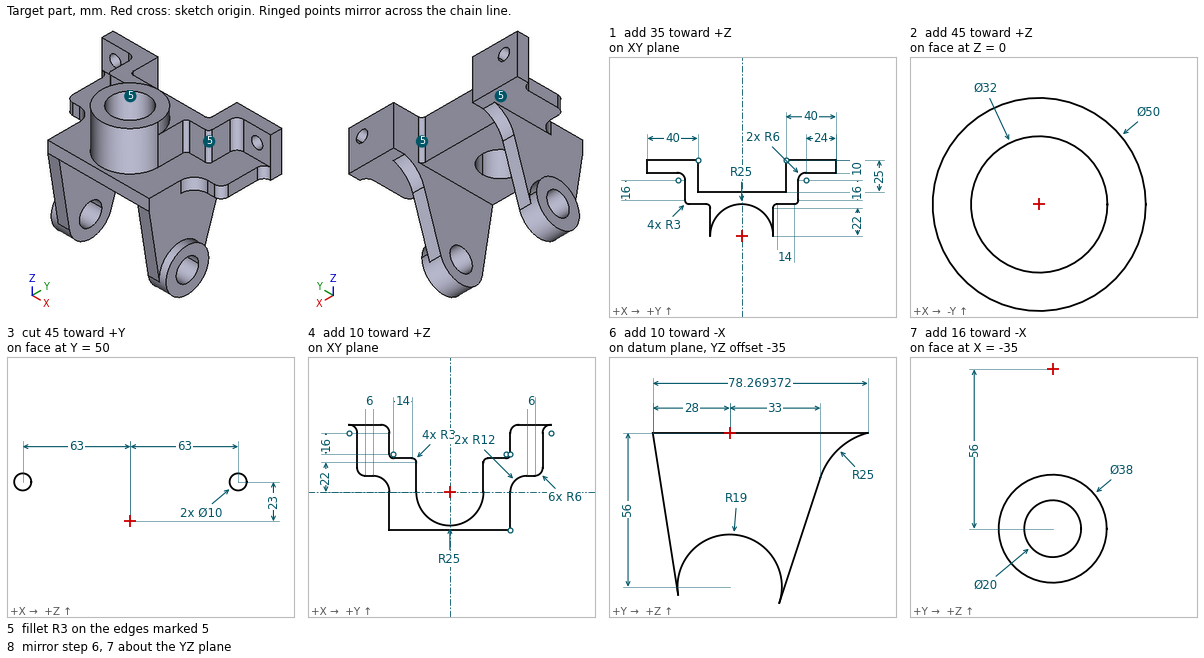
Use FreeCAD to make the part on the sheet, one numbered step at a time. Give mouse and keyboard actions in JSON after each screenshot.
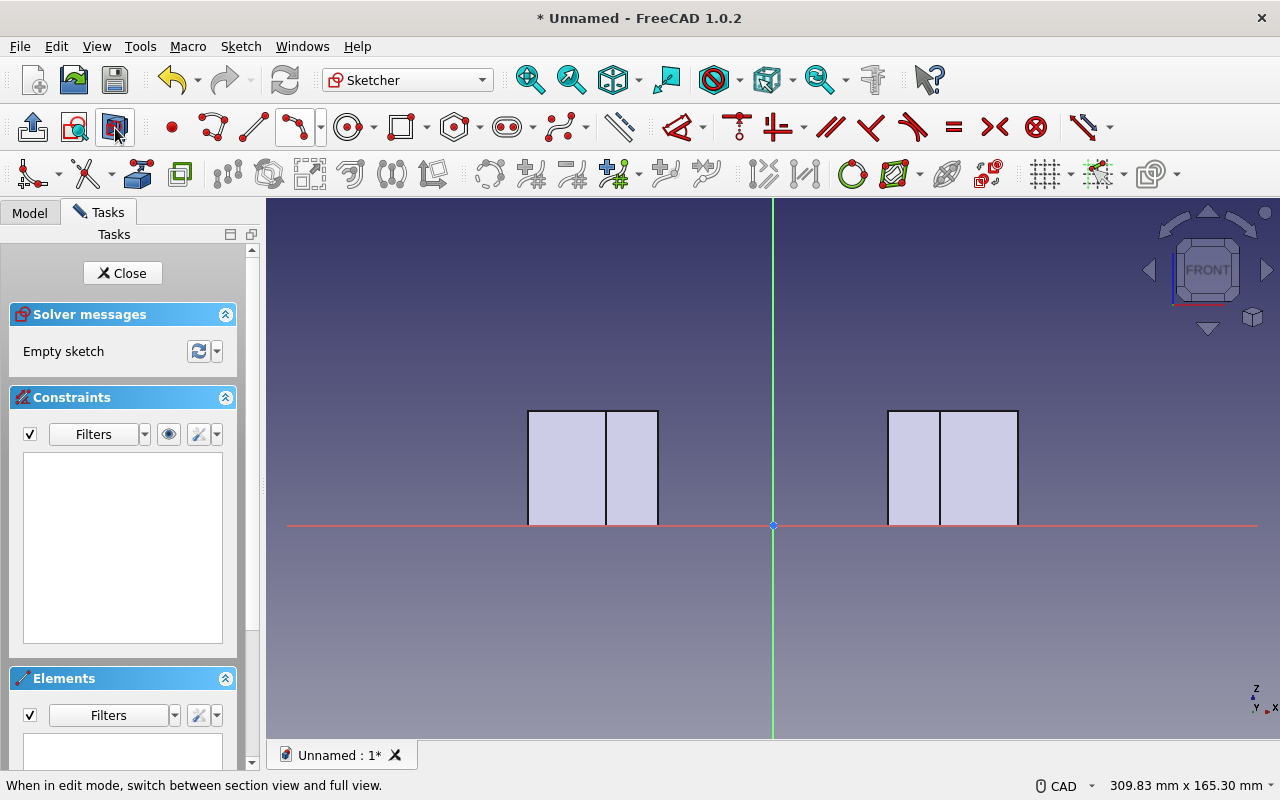
{"action": "left_click", "coordinate": [348, 128]}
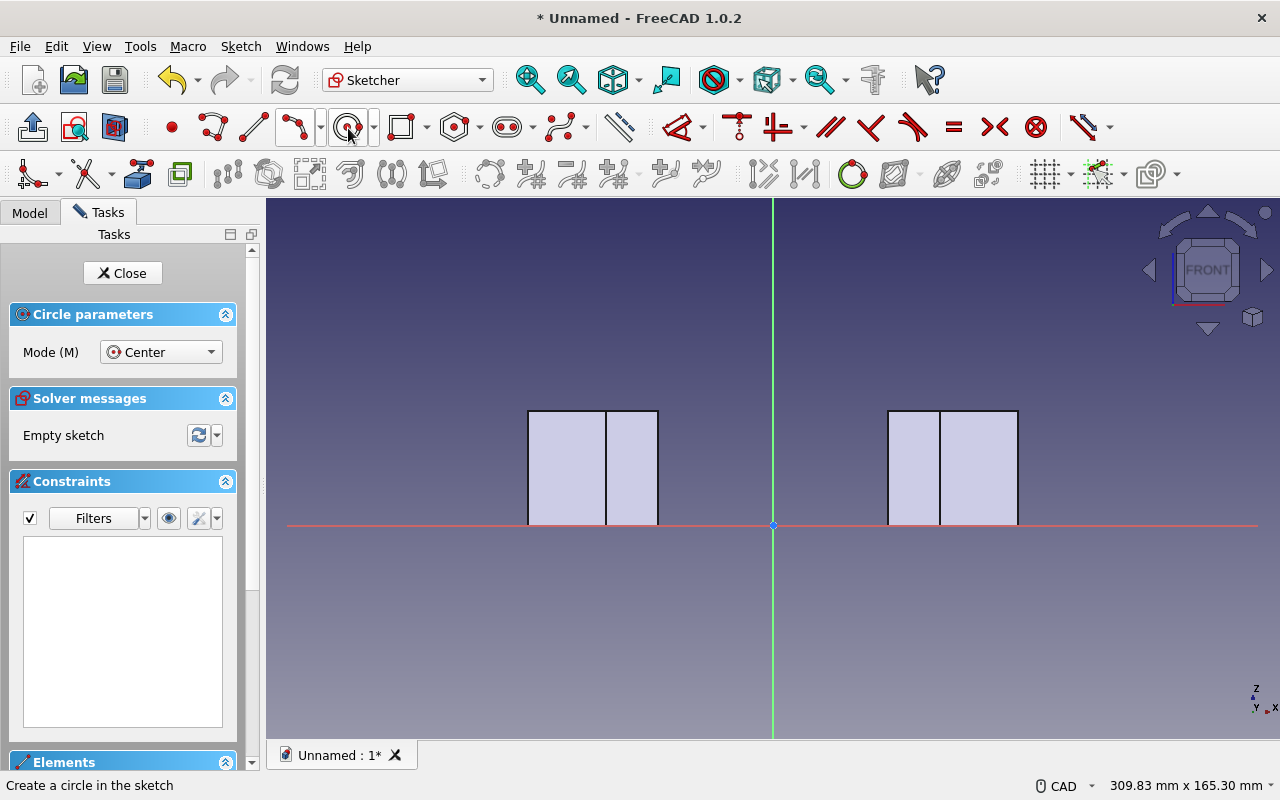
{"action": "scroll", "coordinate": [979, 450], "scroll_direction": "up", "scroll_amount": 2}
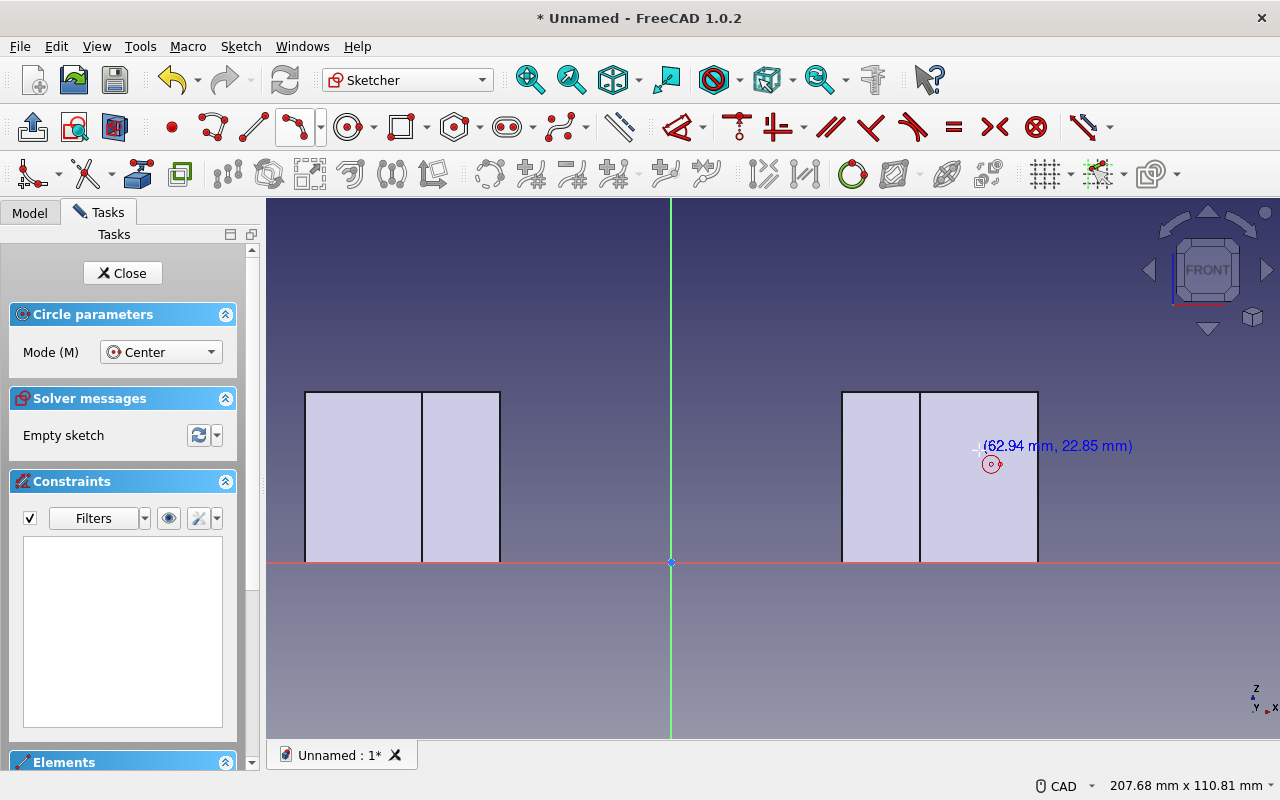
{"action": "left_click", "coordinate": [979, 451]}
{"action": "left_click", "coordinate": [996, 433]}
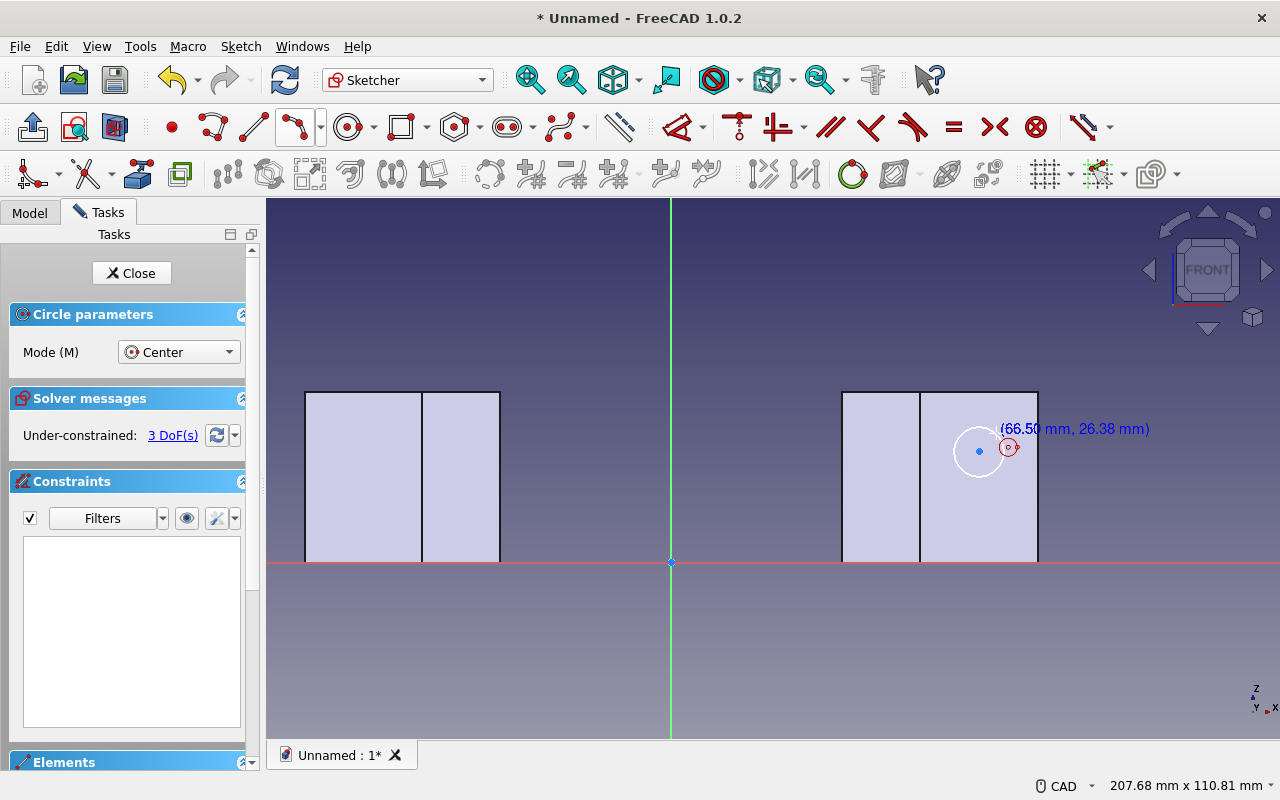
{"action": "left_click", "coordinate": [364, 451]}
{"action": "left_click", "coordinate": [381, 433]}
{"action": "key", "text": "Escape"}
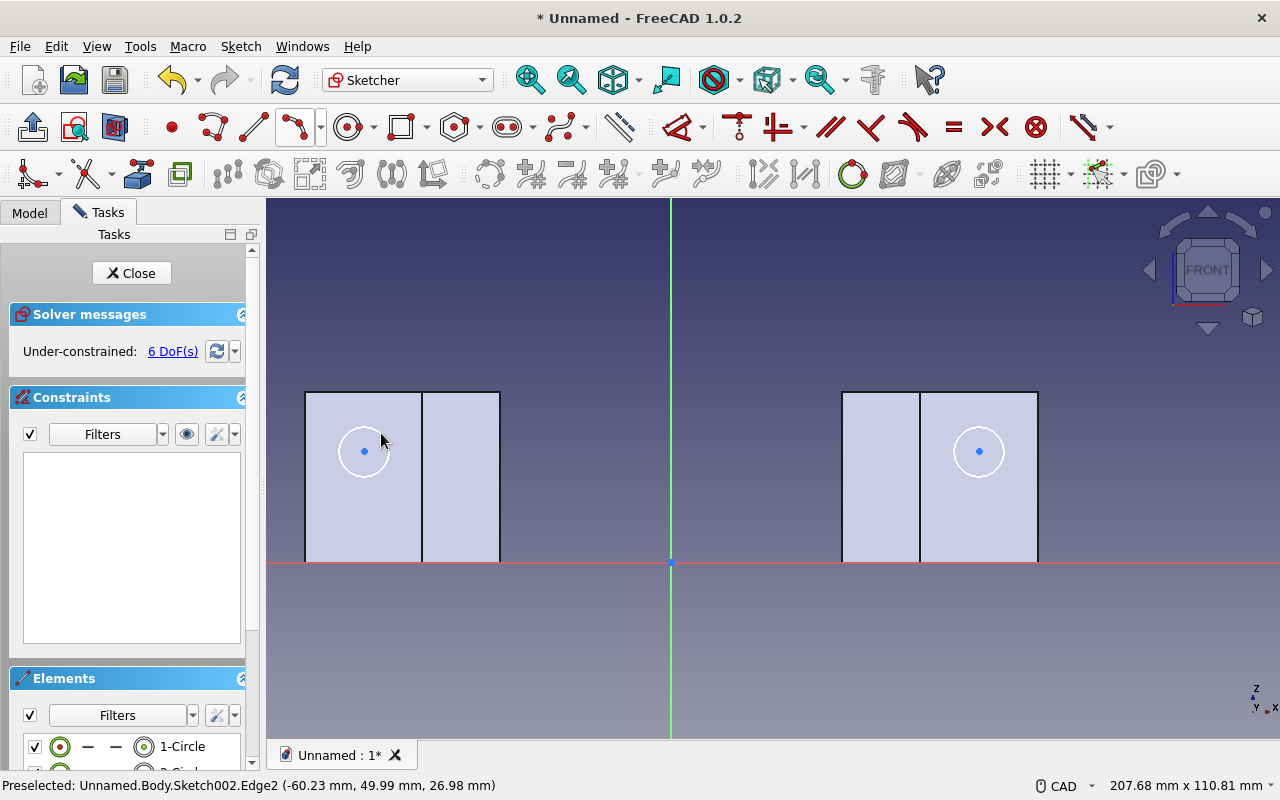
{"action": "left_click", "coordinate": [996, 434]}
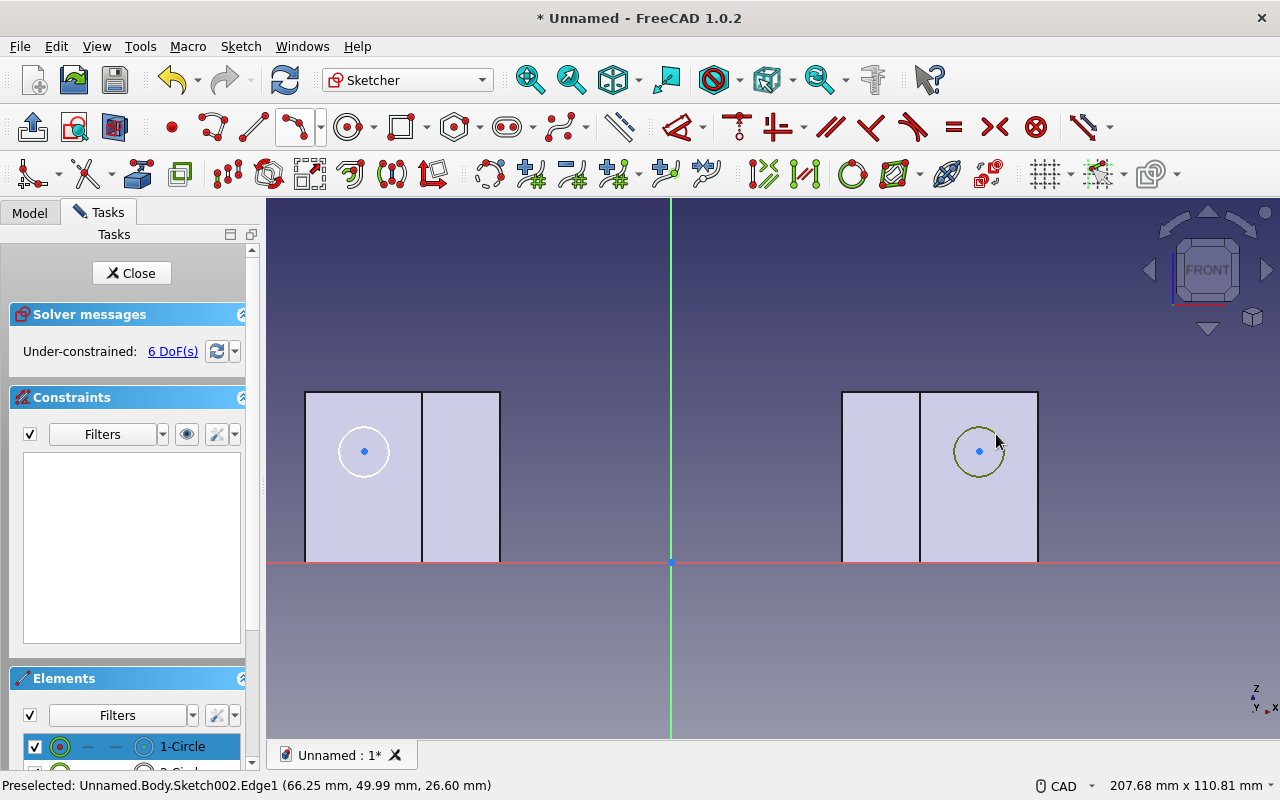
{"action": "left_click", "coordinate": [381, 434]}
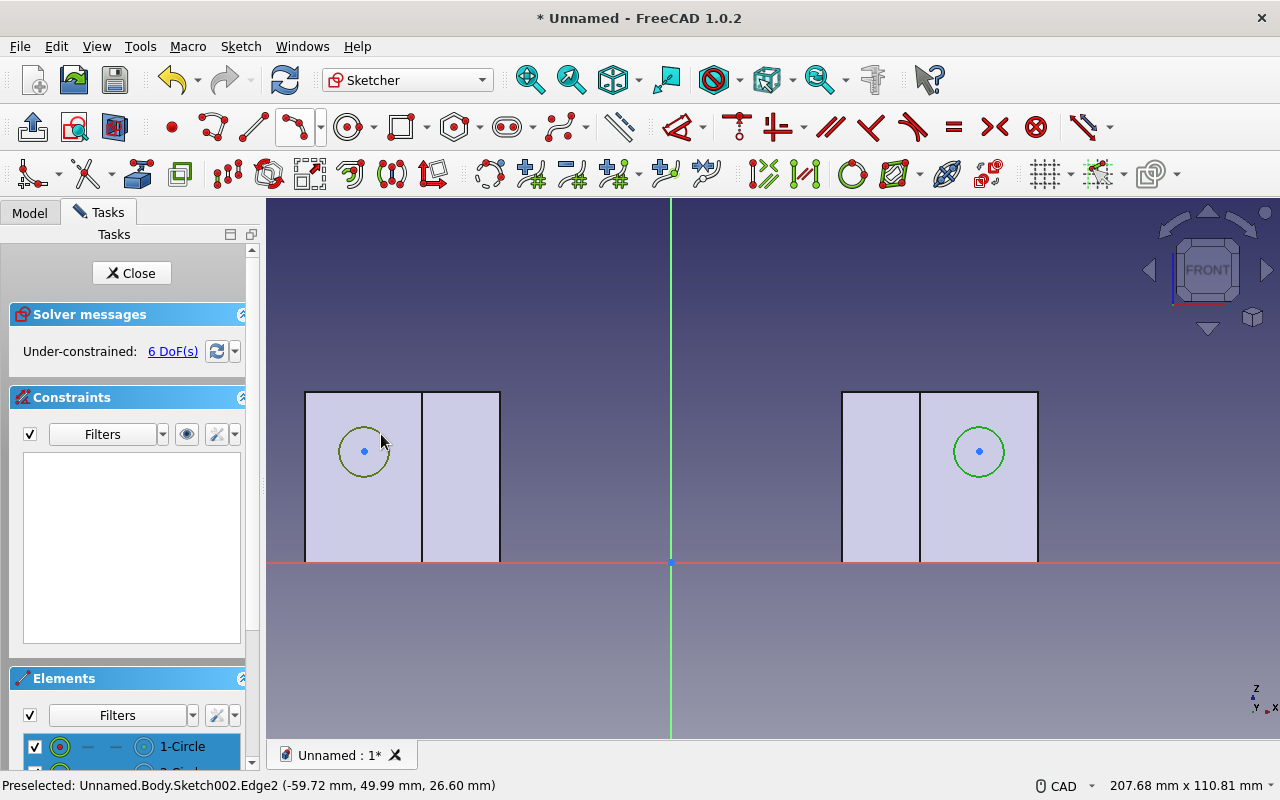
{"action": "left_click", "coordinate": [954, 128]}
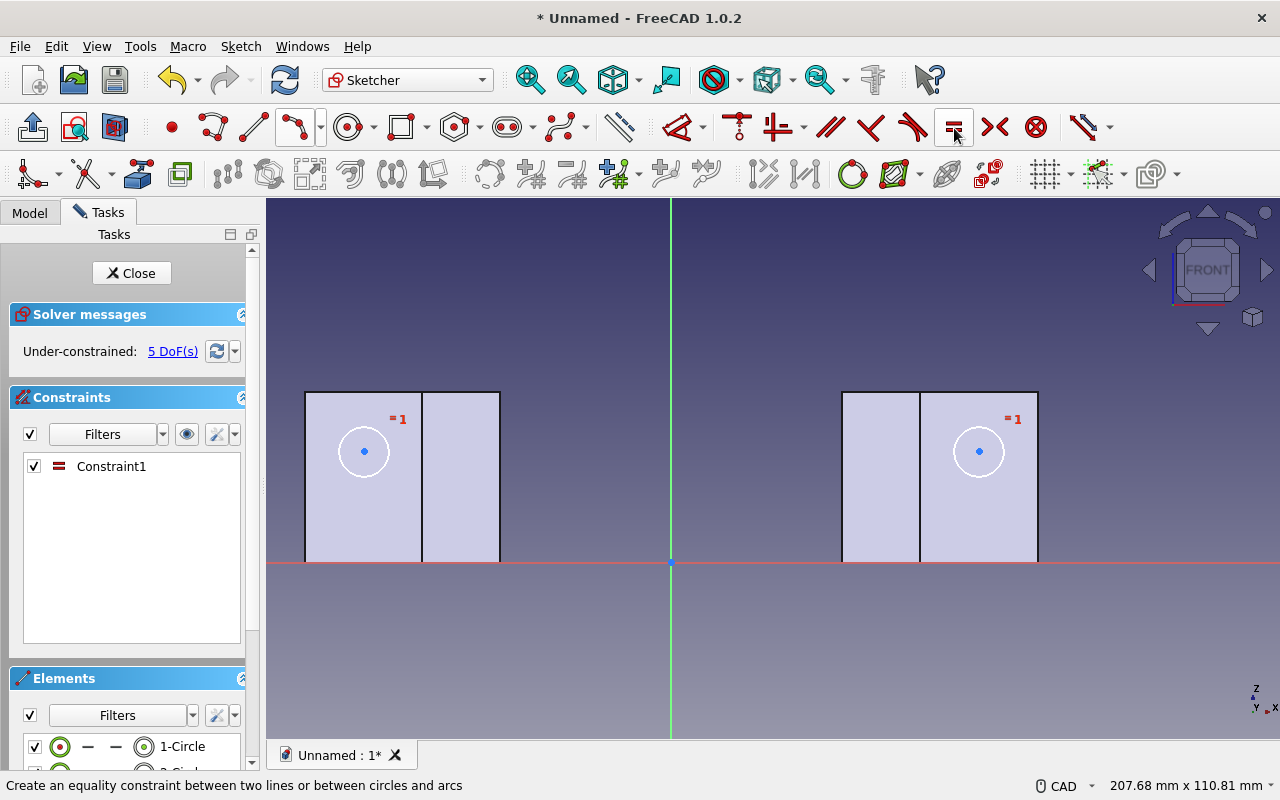
{"action": "left_click", "coordinate": [979, 452]}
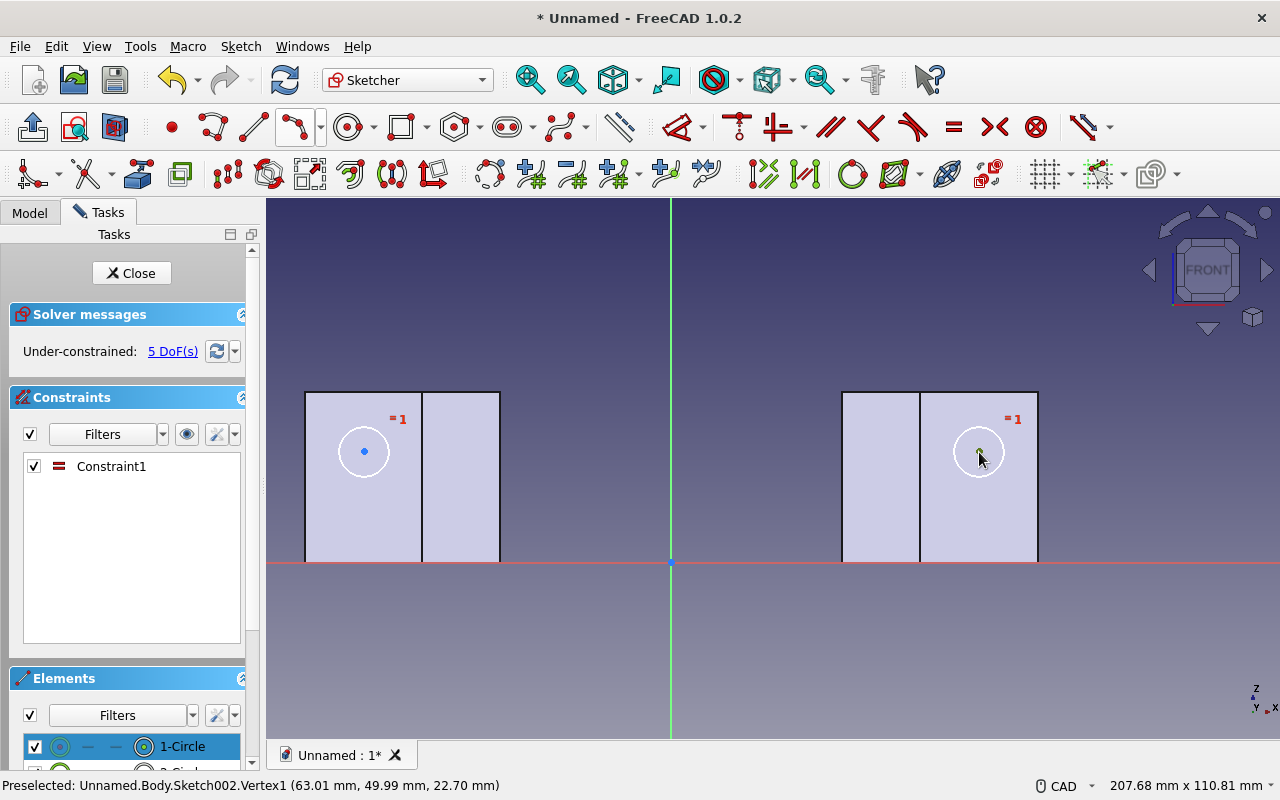
{"action": "left_click", "coordinate": [364, 452]}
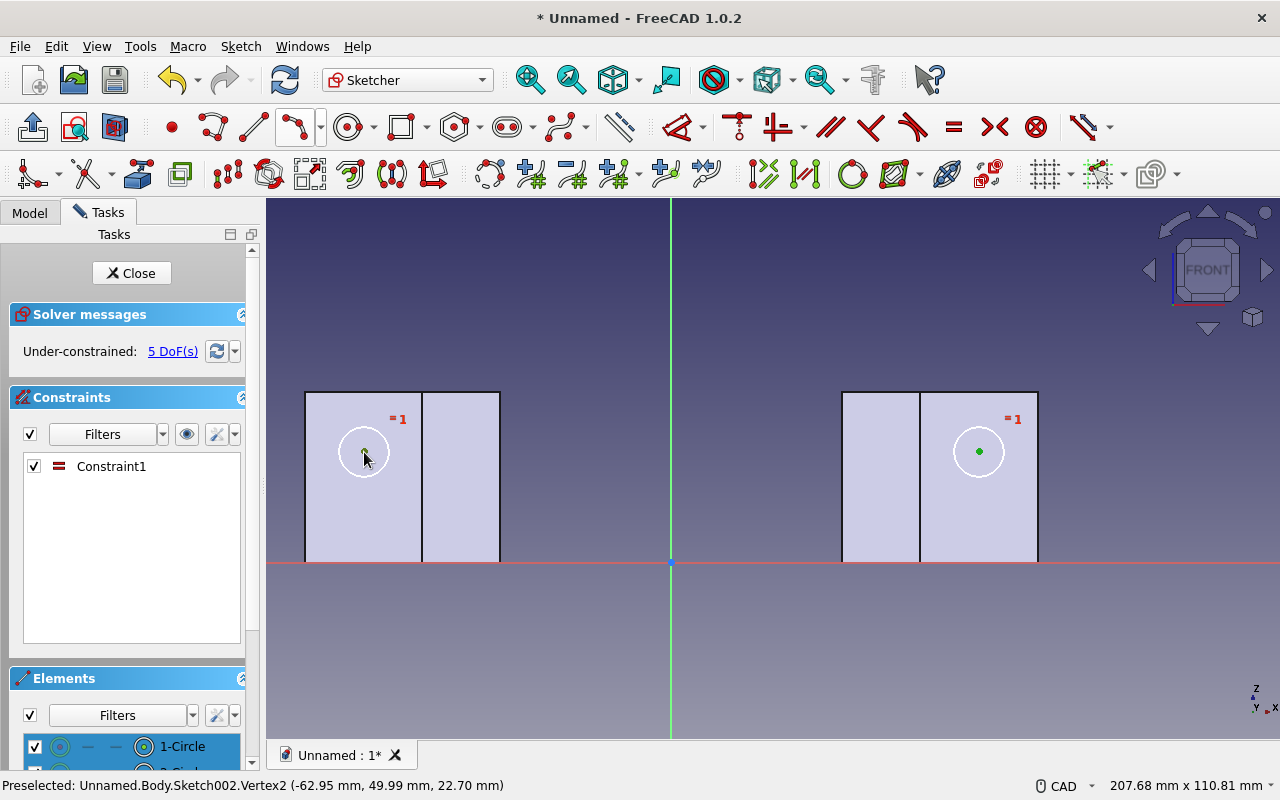
{"action": "left_click", "coordinate": [804, 128]}